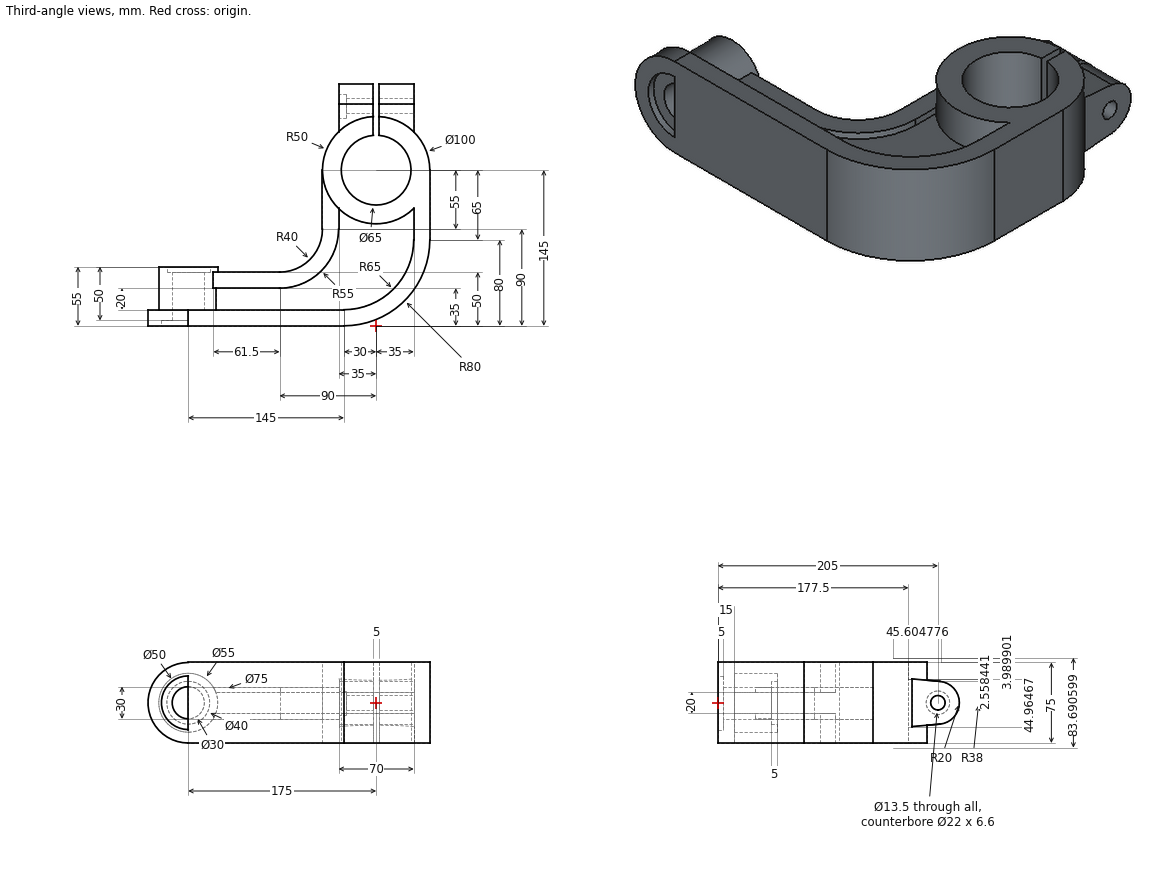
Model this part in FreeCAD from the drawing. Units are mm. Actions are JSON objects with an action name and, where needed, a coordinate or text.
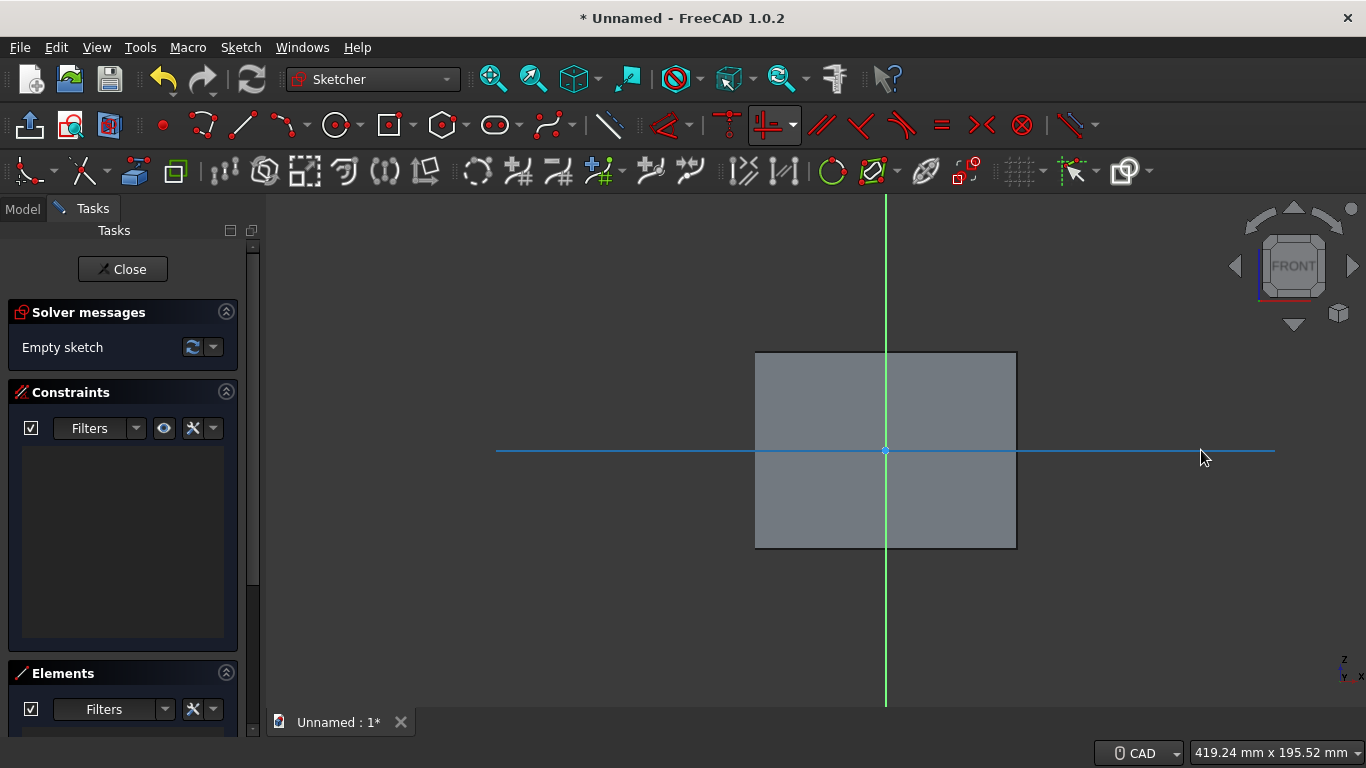
{"action": "scroll", "coordinate": [294, 451], "scroll_direction": "up", "scroll_amount": 2}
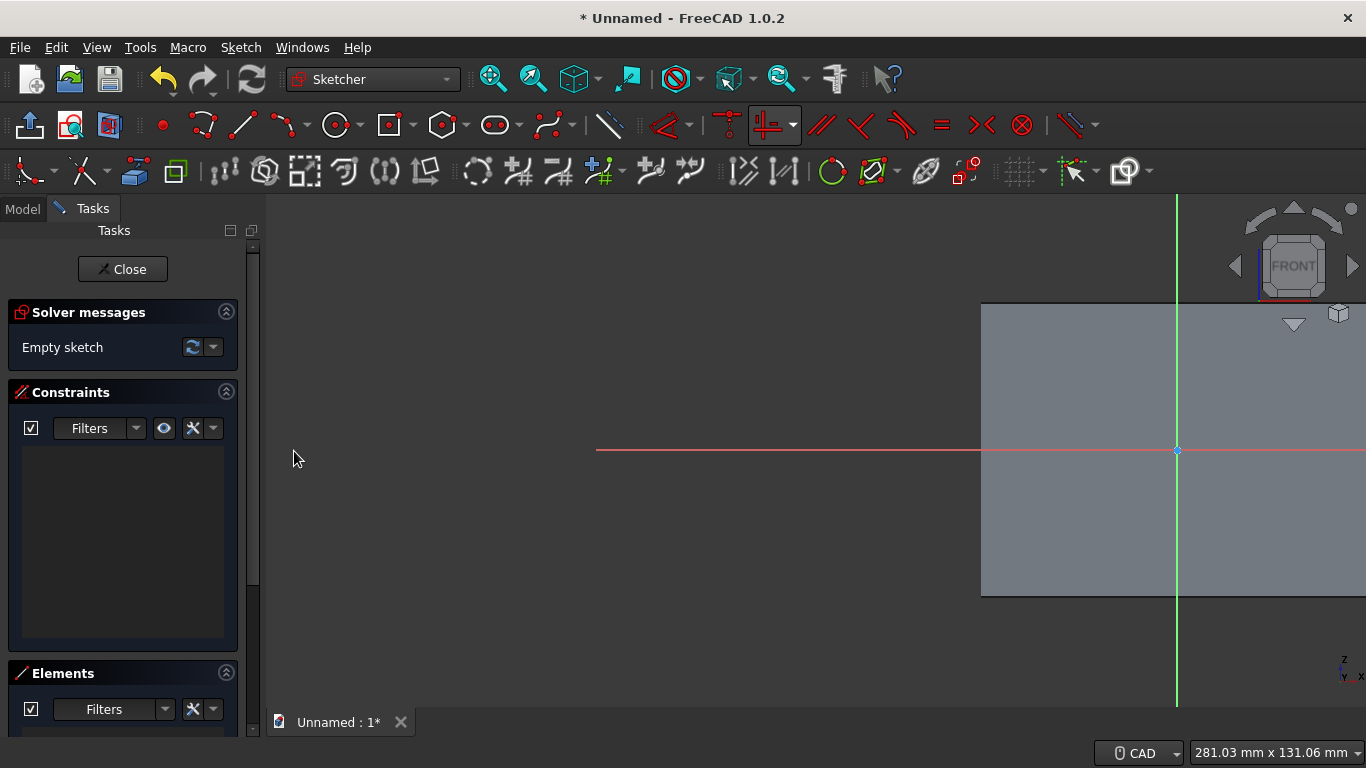
{"action": "key", "text": "g c"}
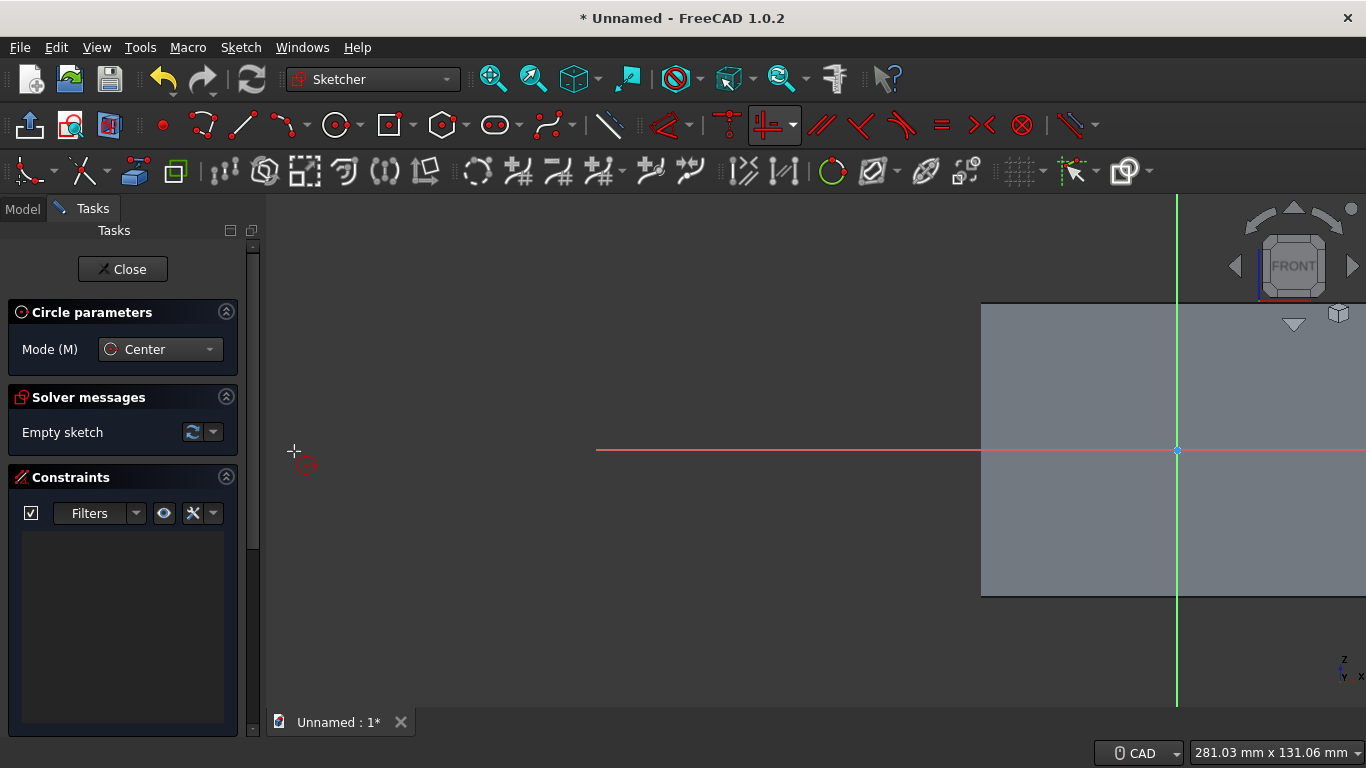
{"action": "left_click", "coordinate": [492, 450]}
{"action": "left_click", "coordinate": [596, 346]}
{"action": "key", "text": "Escape"}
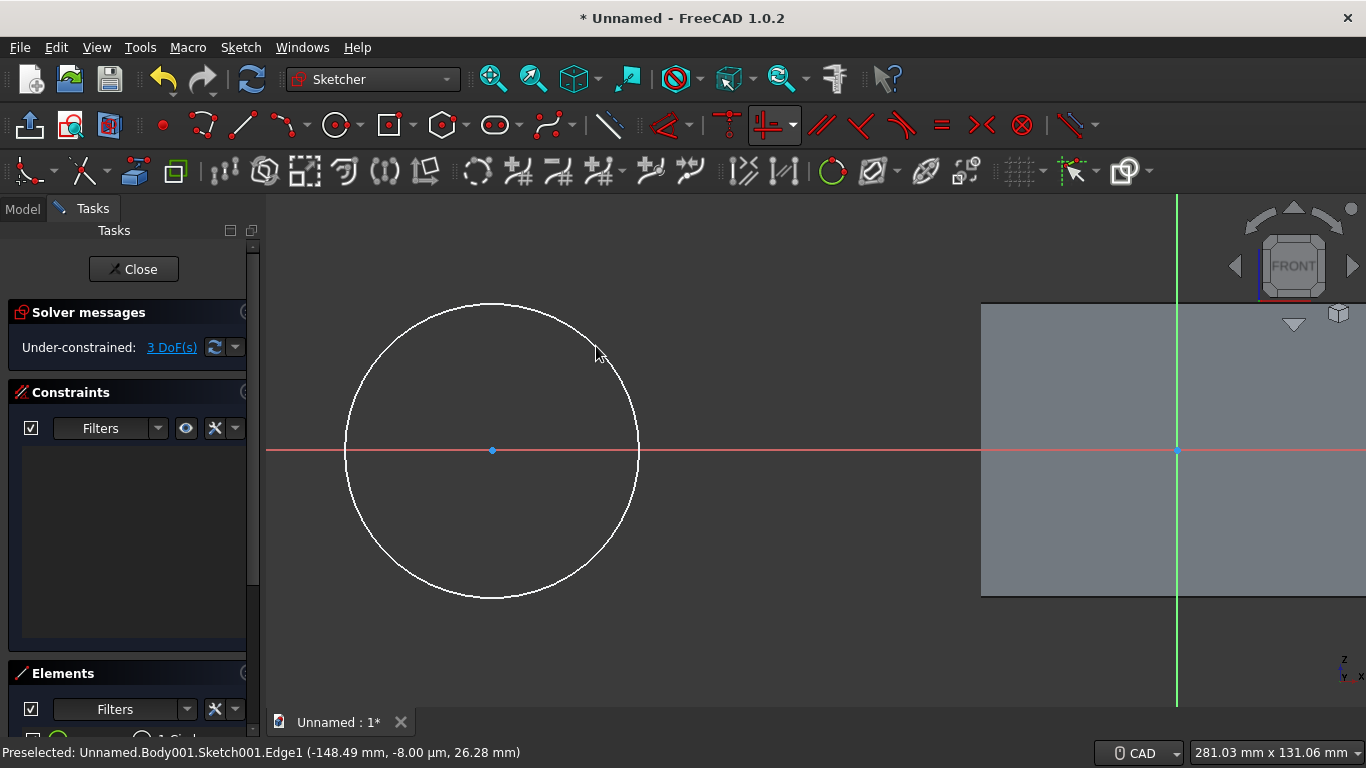
{"action": "left_click", "coordinate": [492, 451]}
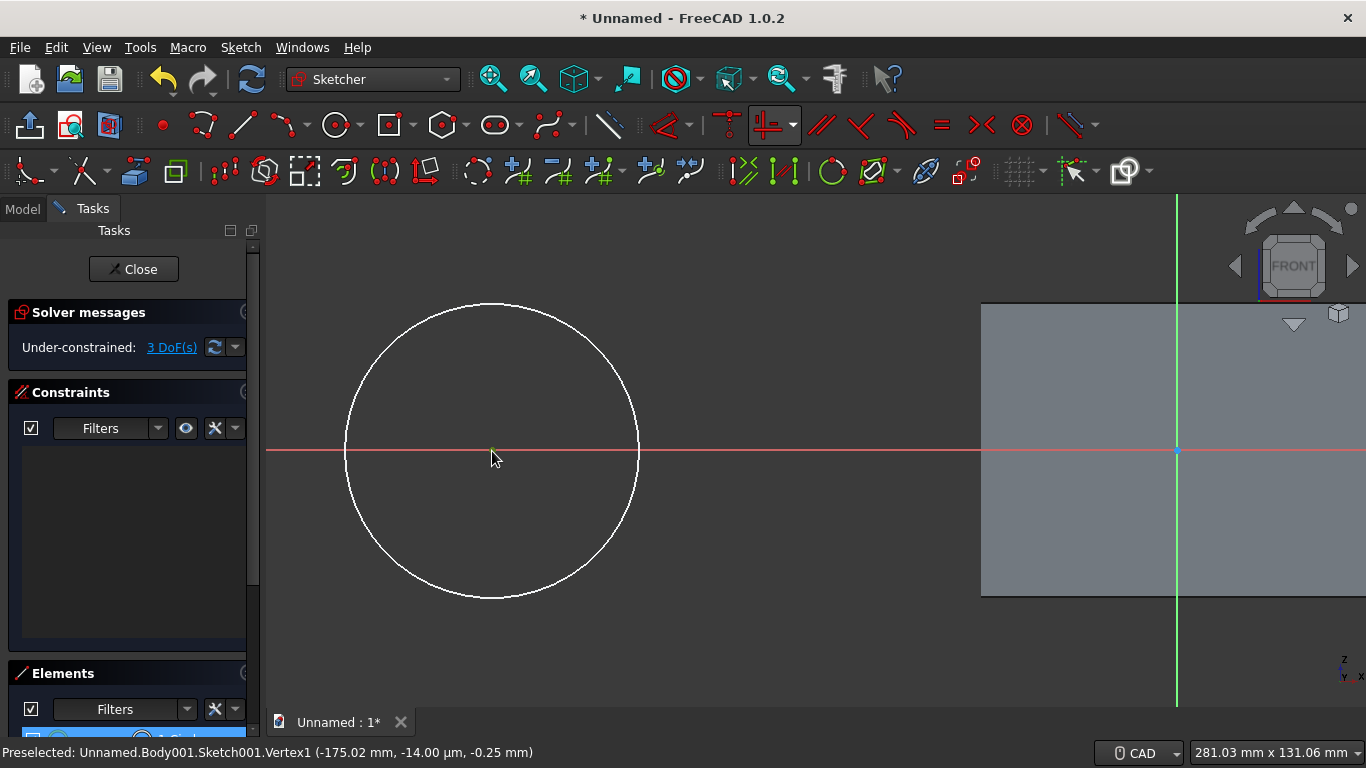
{"action": "left_click", "coordinate": [424, 450]}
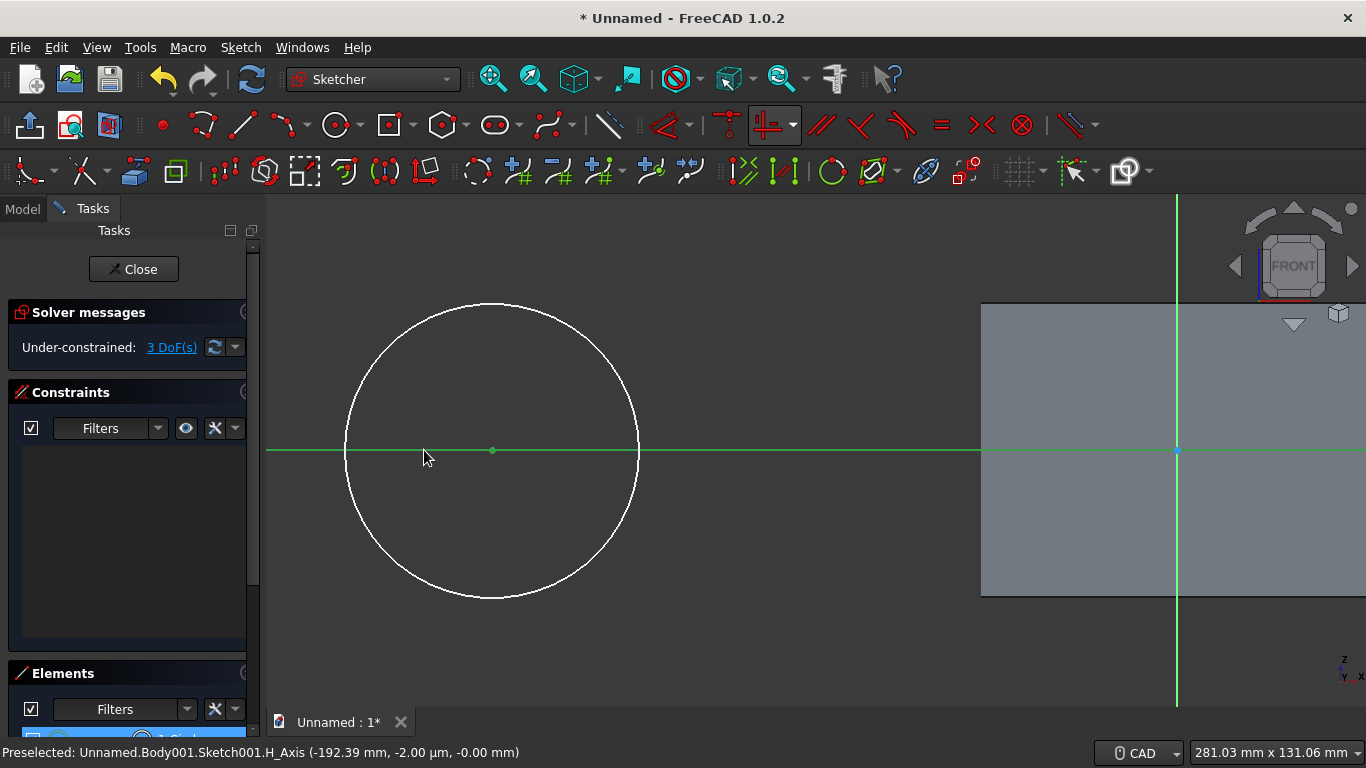
{"action": "key", "text": "c"}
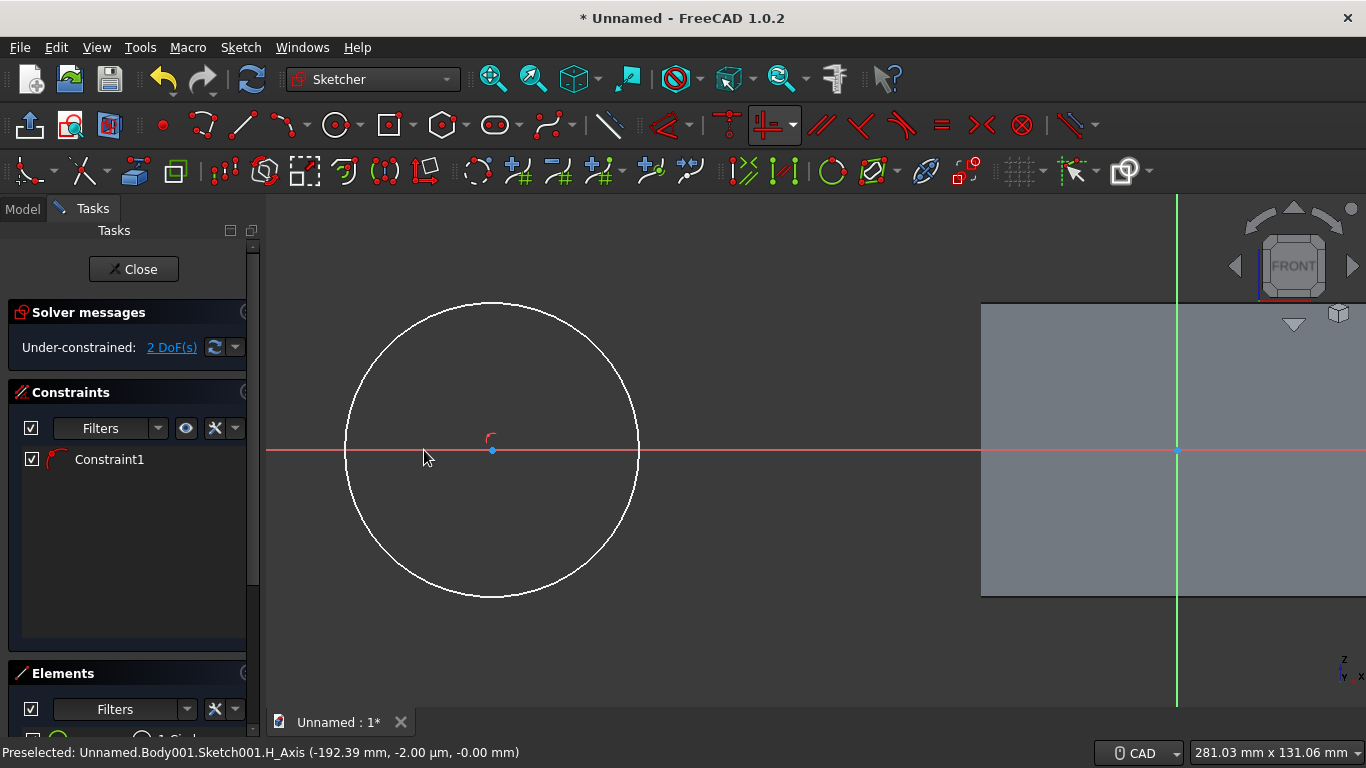
{"action": "left_click", "coordinate": [664, 126]}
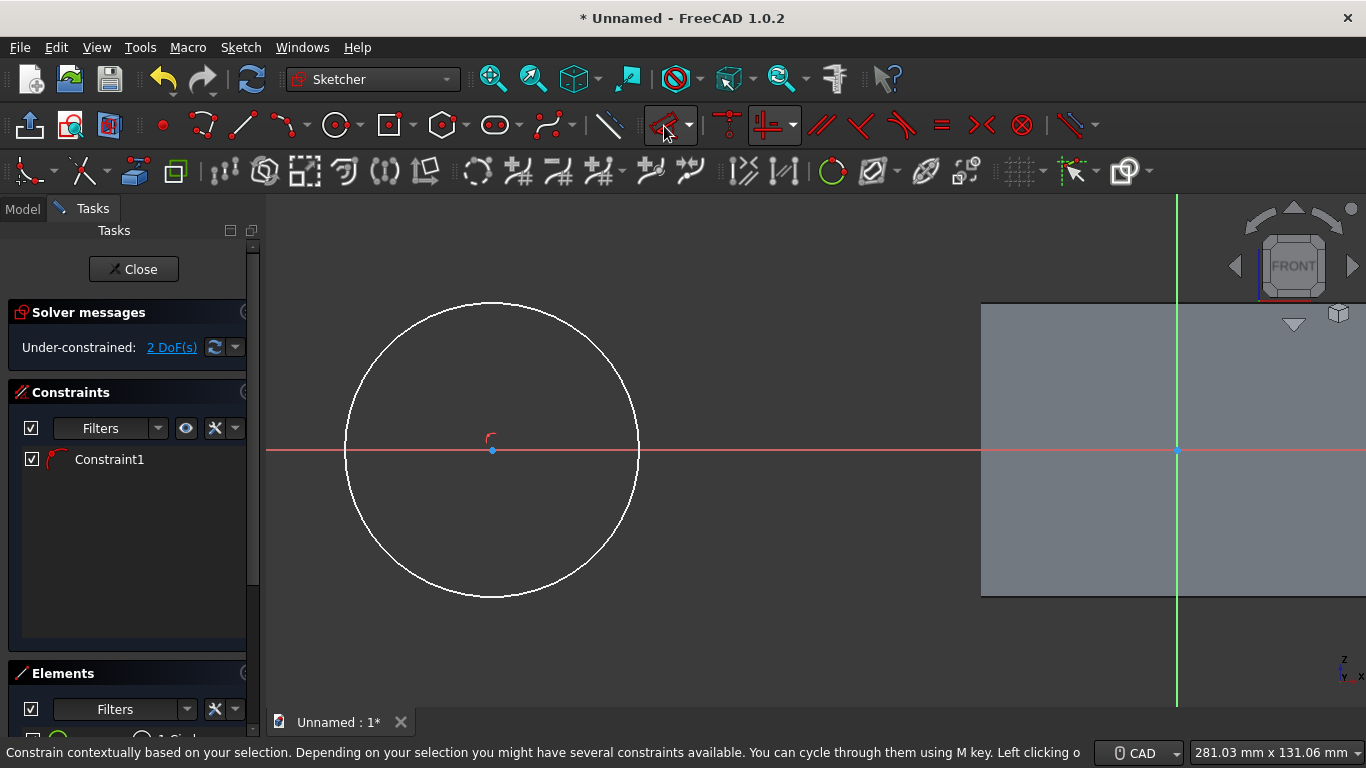
{"action": "left_click", "coordinate": [596, 346]}
{"action": "left_click", "coordinate": [619, 323]}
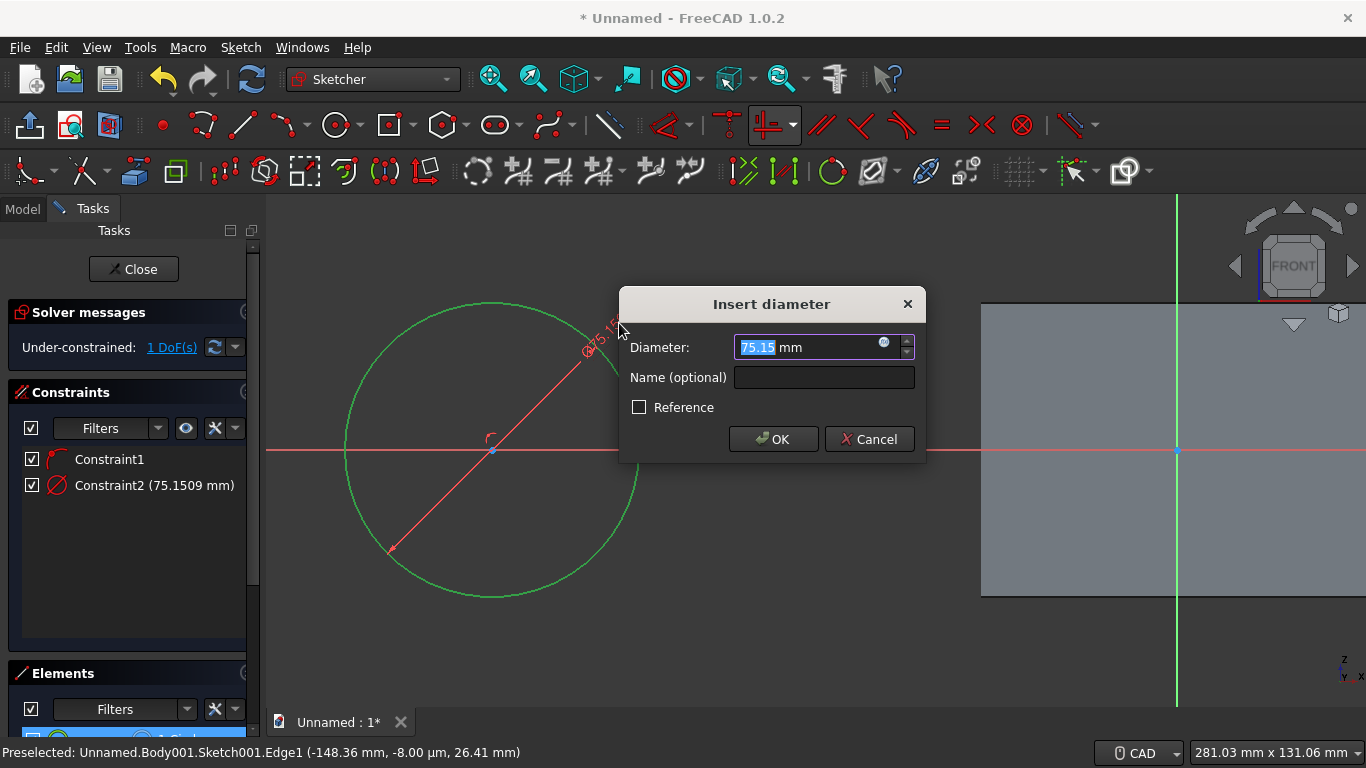
{"action": "type", "text": "75"}
{"action": "key", "text": "Return"}